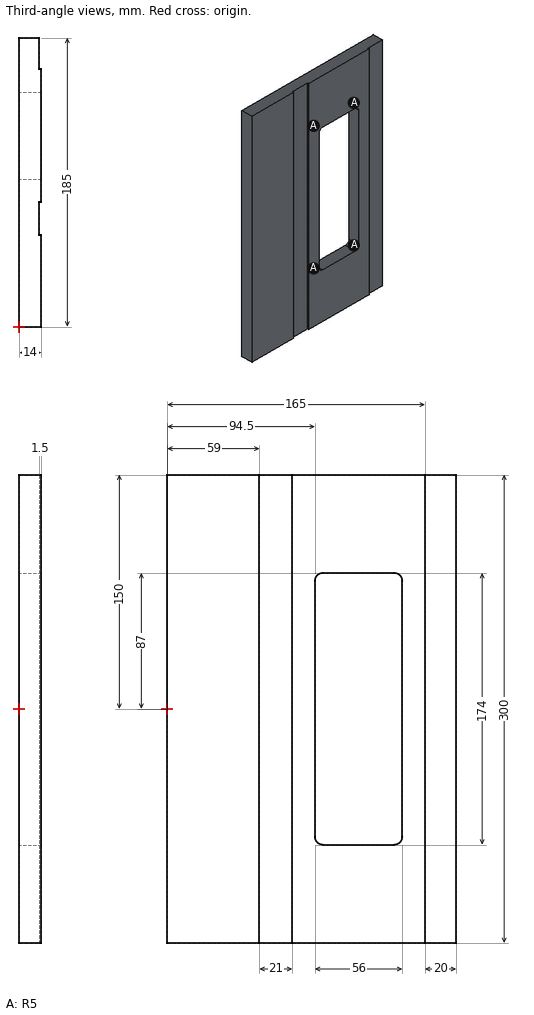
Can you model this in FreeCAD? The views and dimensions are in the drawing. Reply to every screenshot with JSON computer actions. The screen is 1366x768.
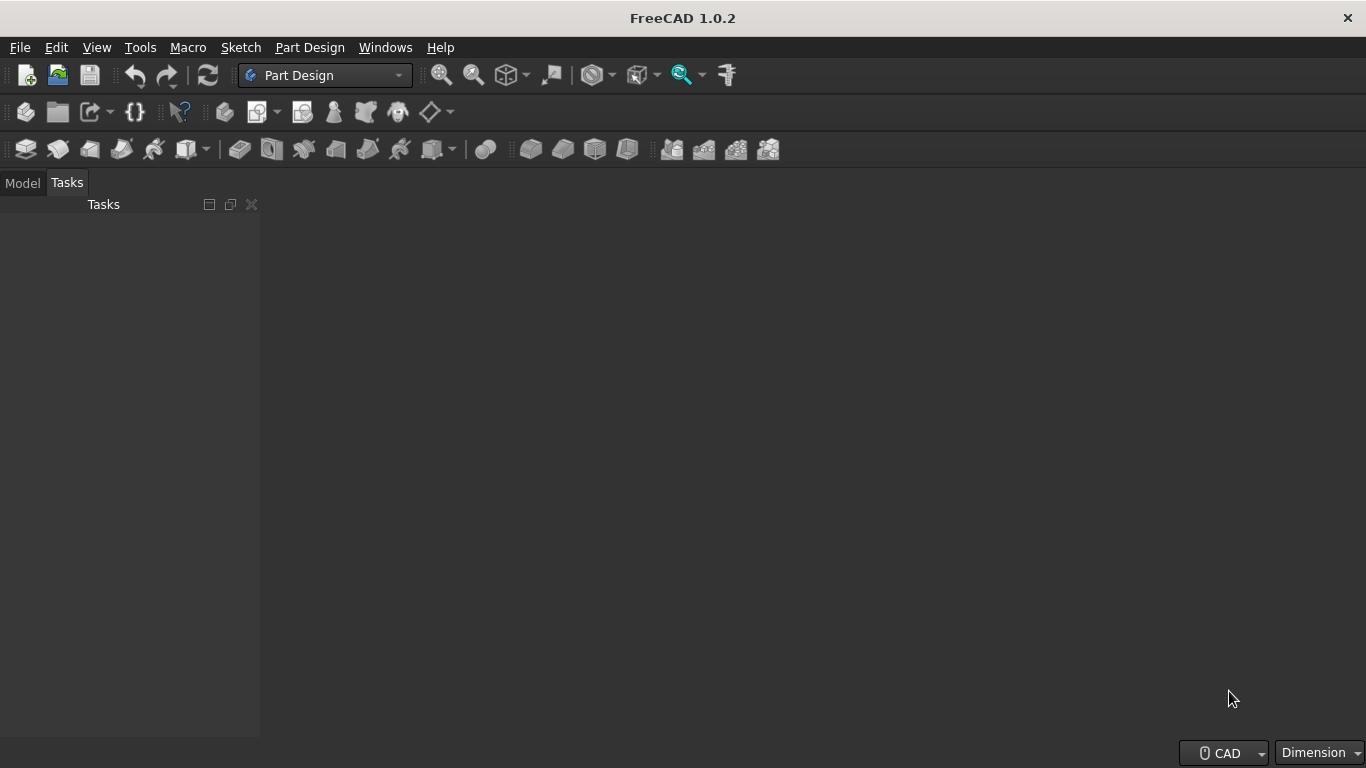
{"action": "left_click", "coordinate": [26, 76]}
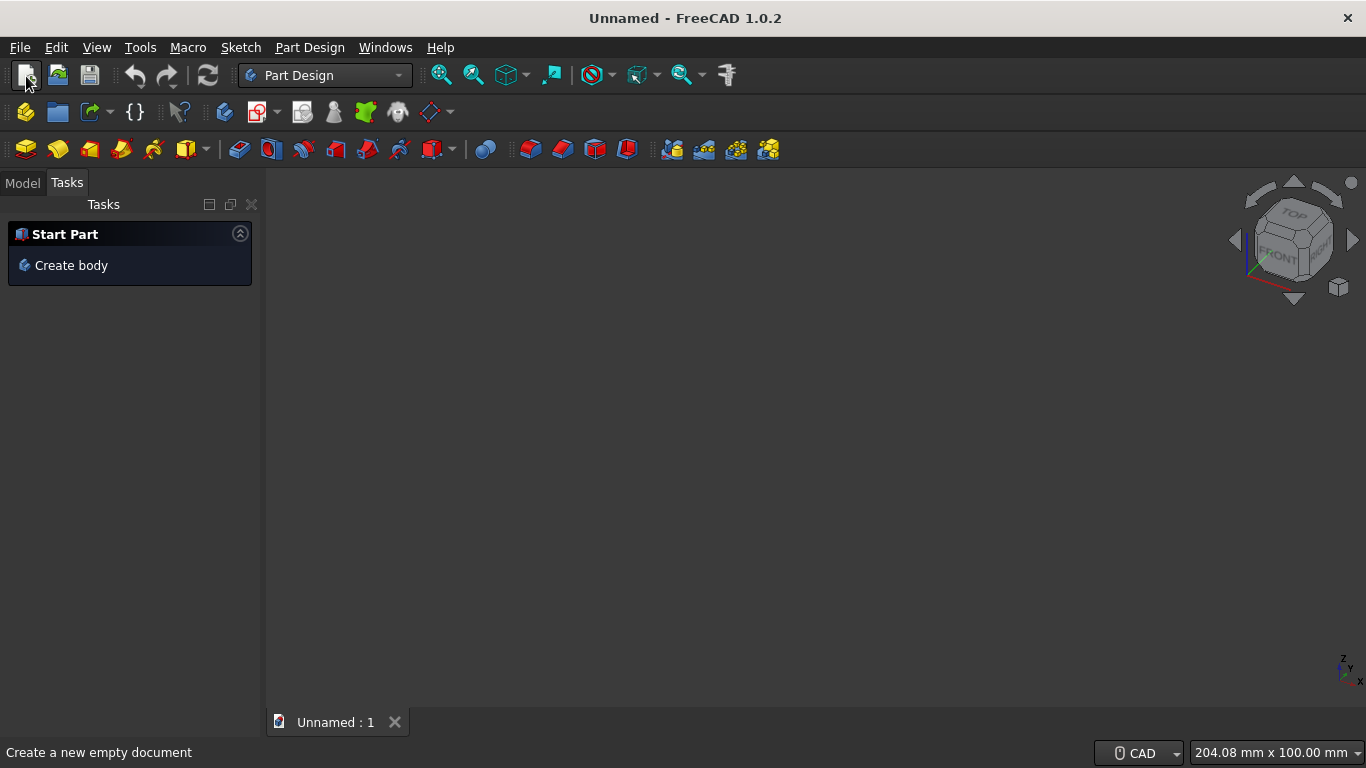
{"action": "left_click", "coordinate": [258, 112]}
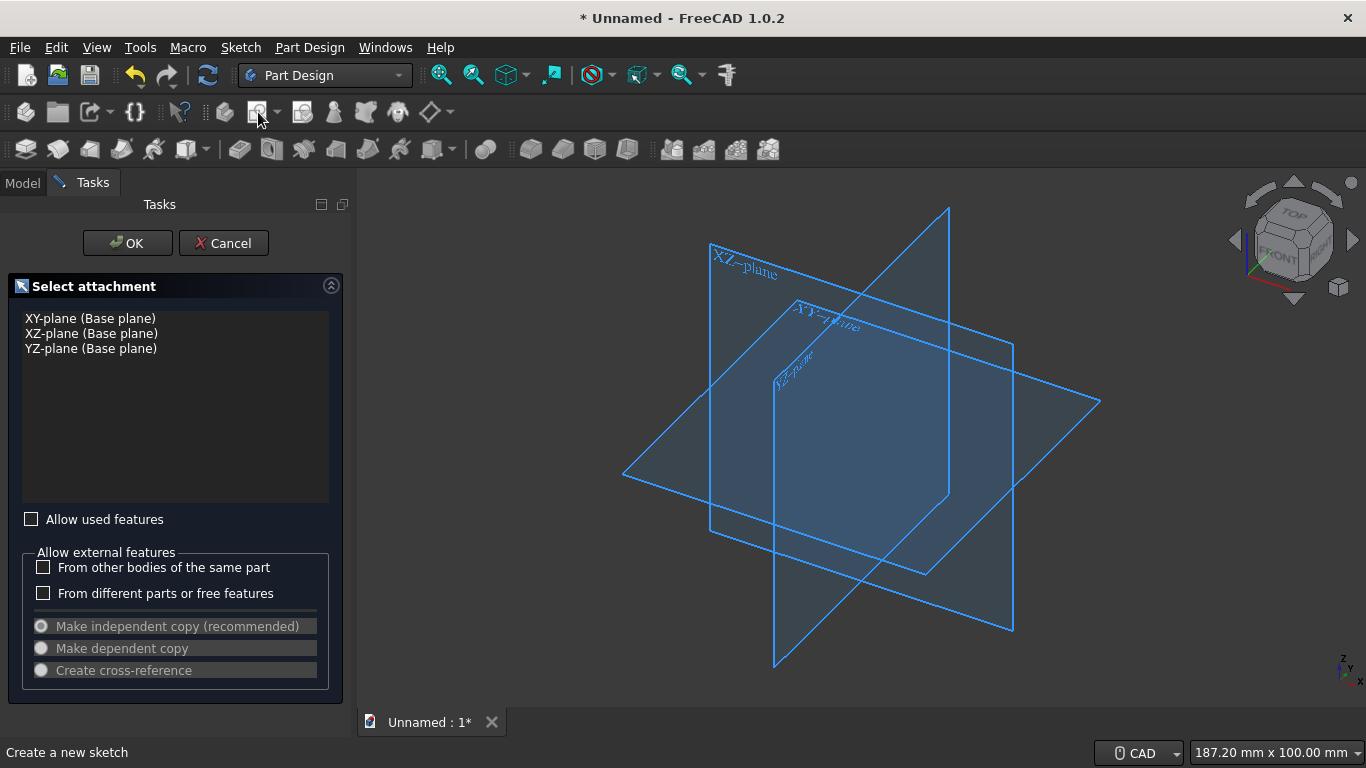
{"action": "left_click", "coordinate": [82, 318]}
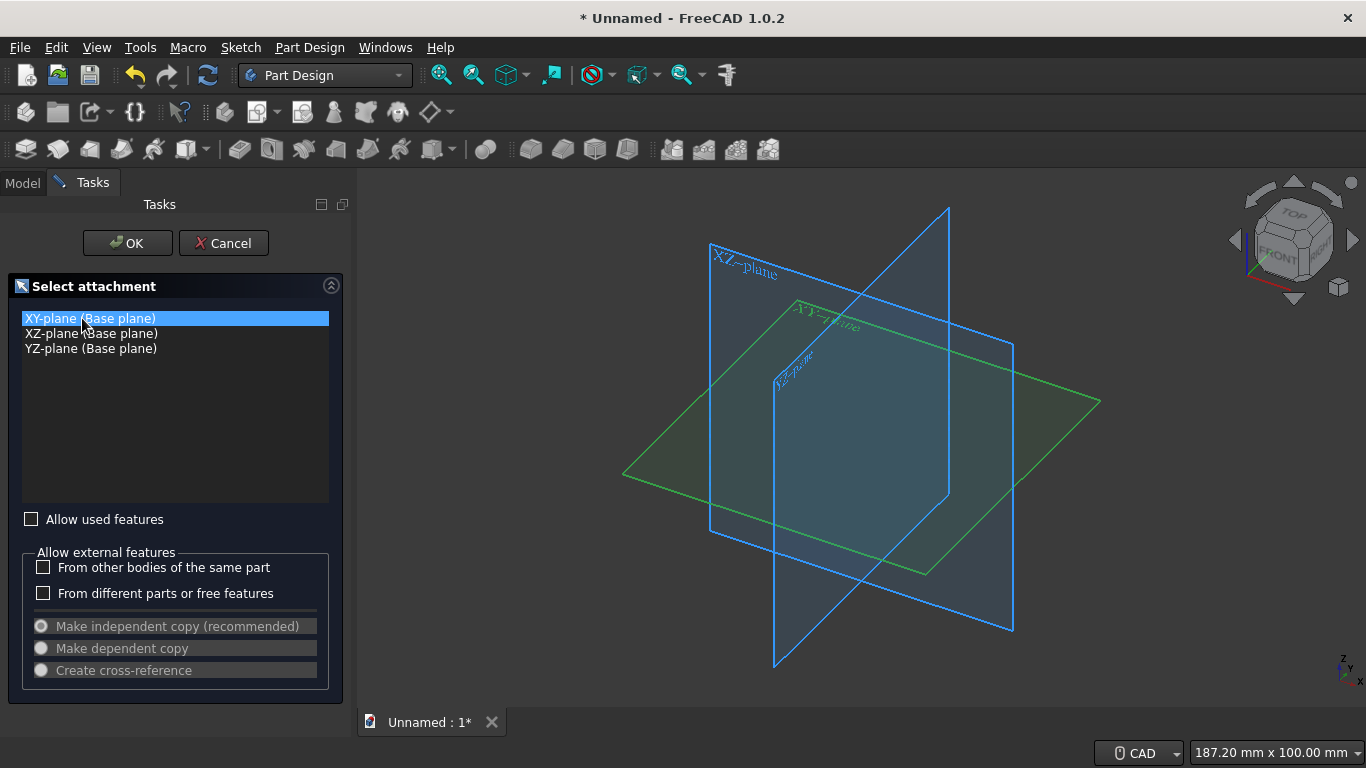
{"action": "left_click", "coordinate": [128, 243]}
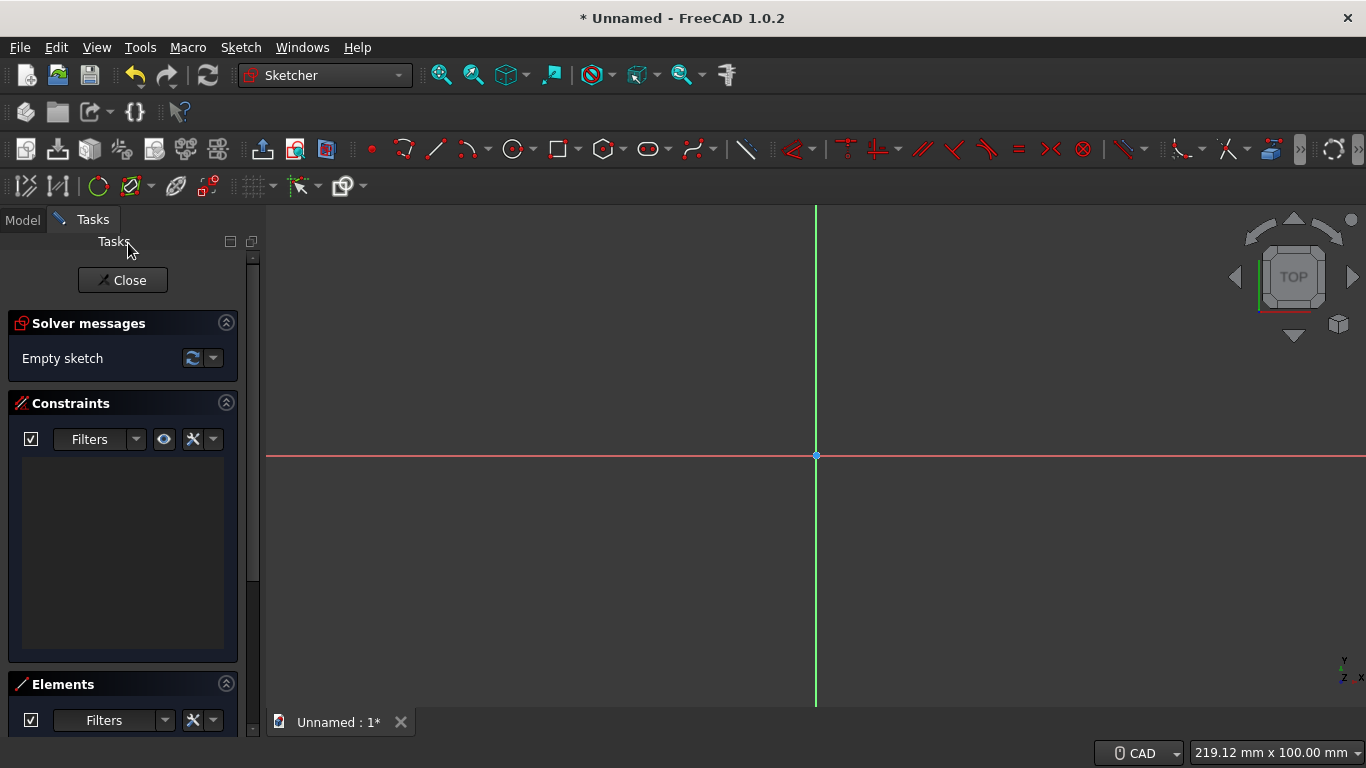
{"action": "scroll", "coordinate": [703, 656], "scroll_direction": "down", "scroll_amount": 6}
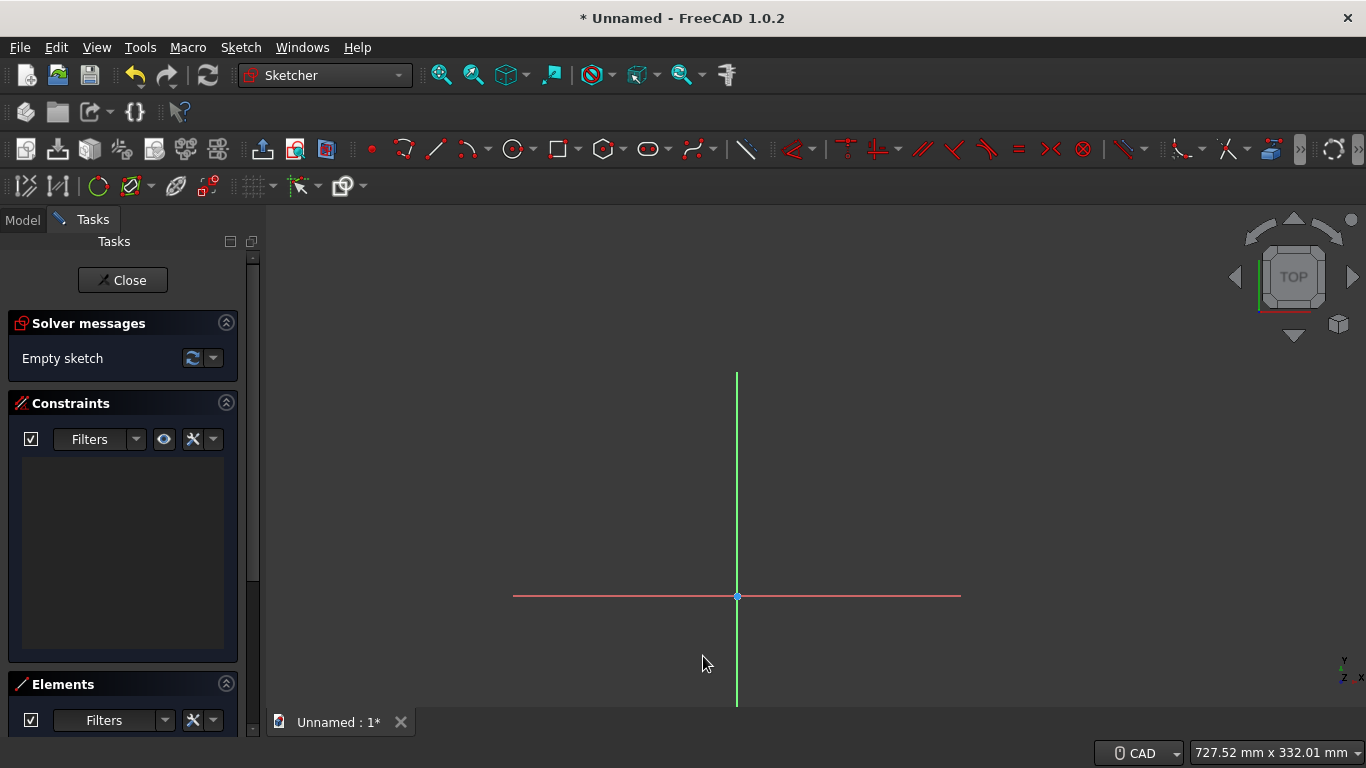
{"action": "left_click", "coordinate": [558, 150]}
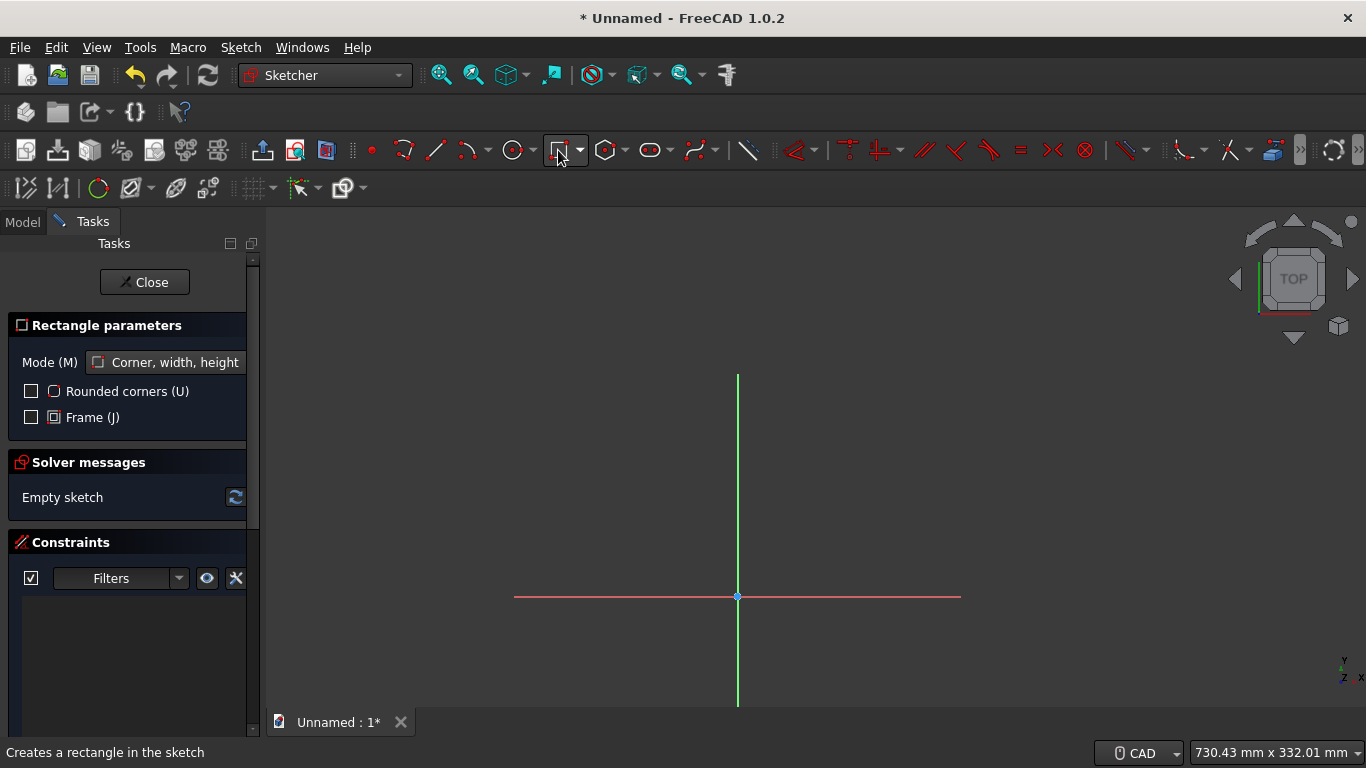
{"action": "left_click", "coordinate": [738, 597]}
{"action": "left_click", "coordinate": [759, 318]}
{"action": "key", "text": "Escape"}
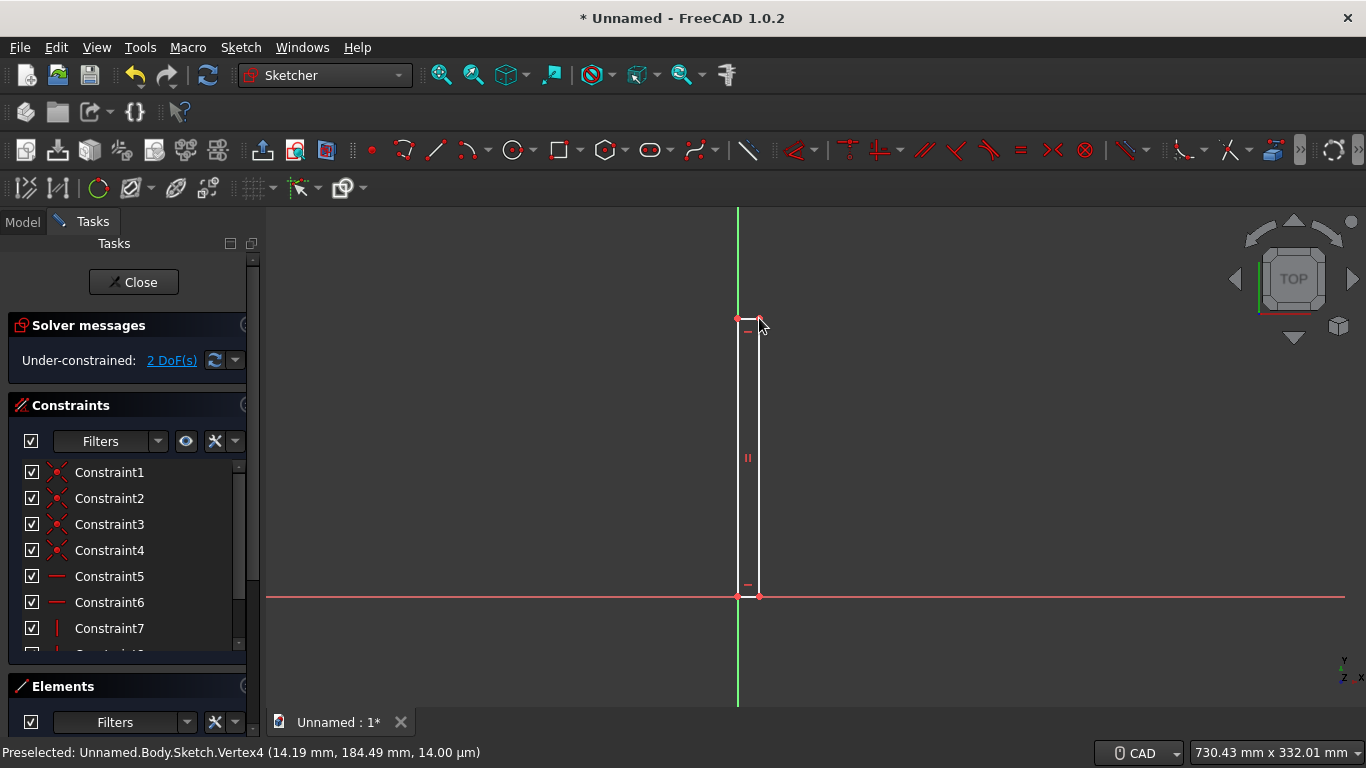
{"action": "left_click", "coordinate": [794, 150]}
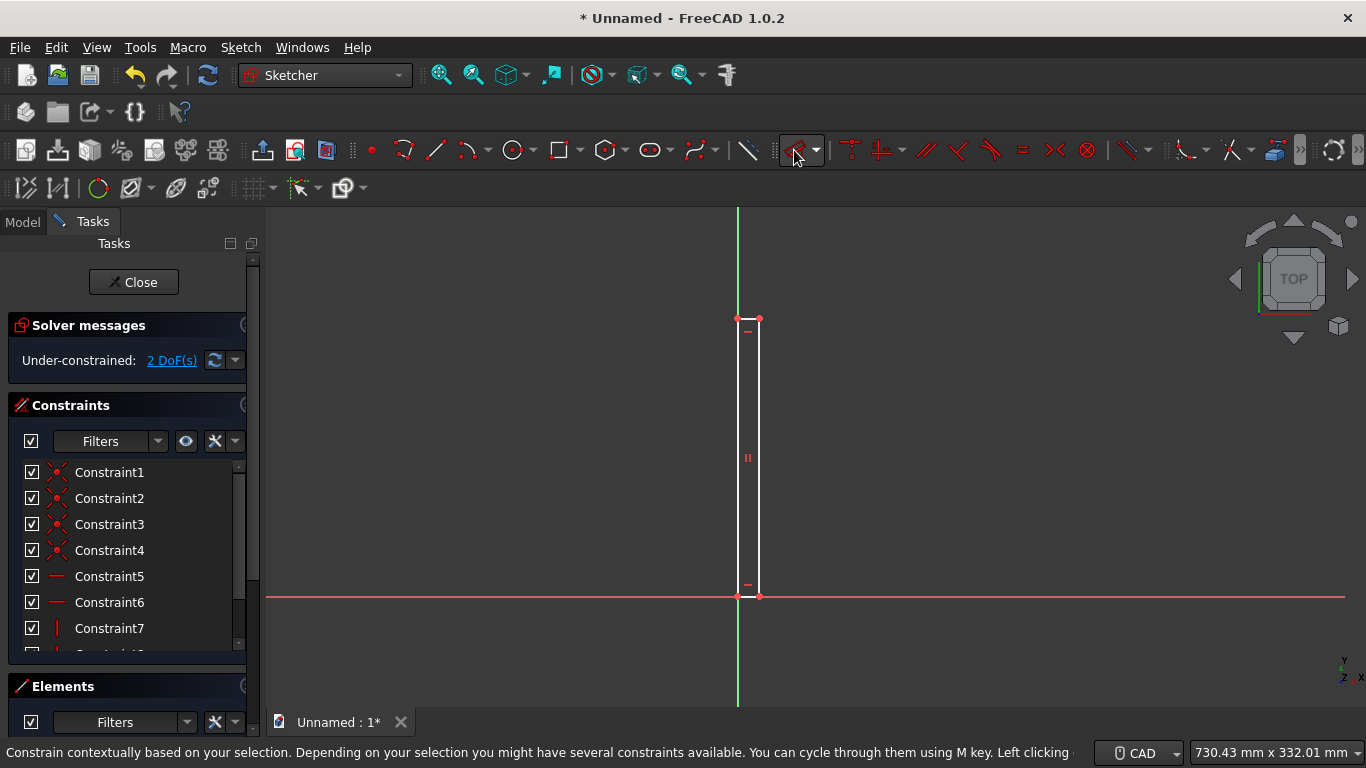
{"action": "scroll", "coordinate": [748, 597], "scroll_direction": "up", "scroll_amount": 4}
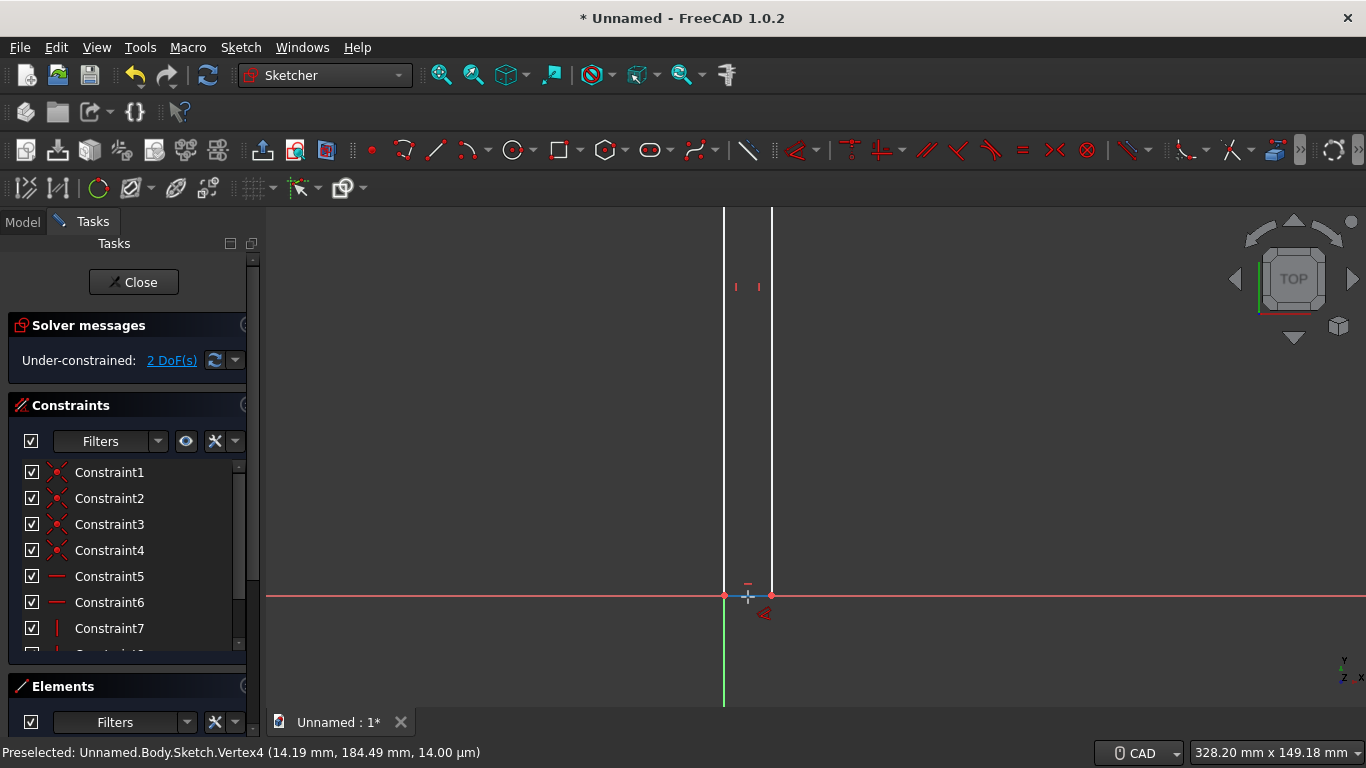
{"action": "left_click", "coordinate": [748, 596]}
{"action": "left_click", "coordinate": [748, 630]}